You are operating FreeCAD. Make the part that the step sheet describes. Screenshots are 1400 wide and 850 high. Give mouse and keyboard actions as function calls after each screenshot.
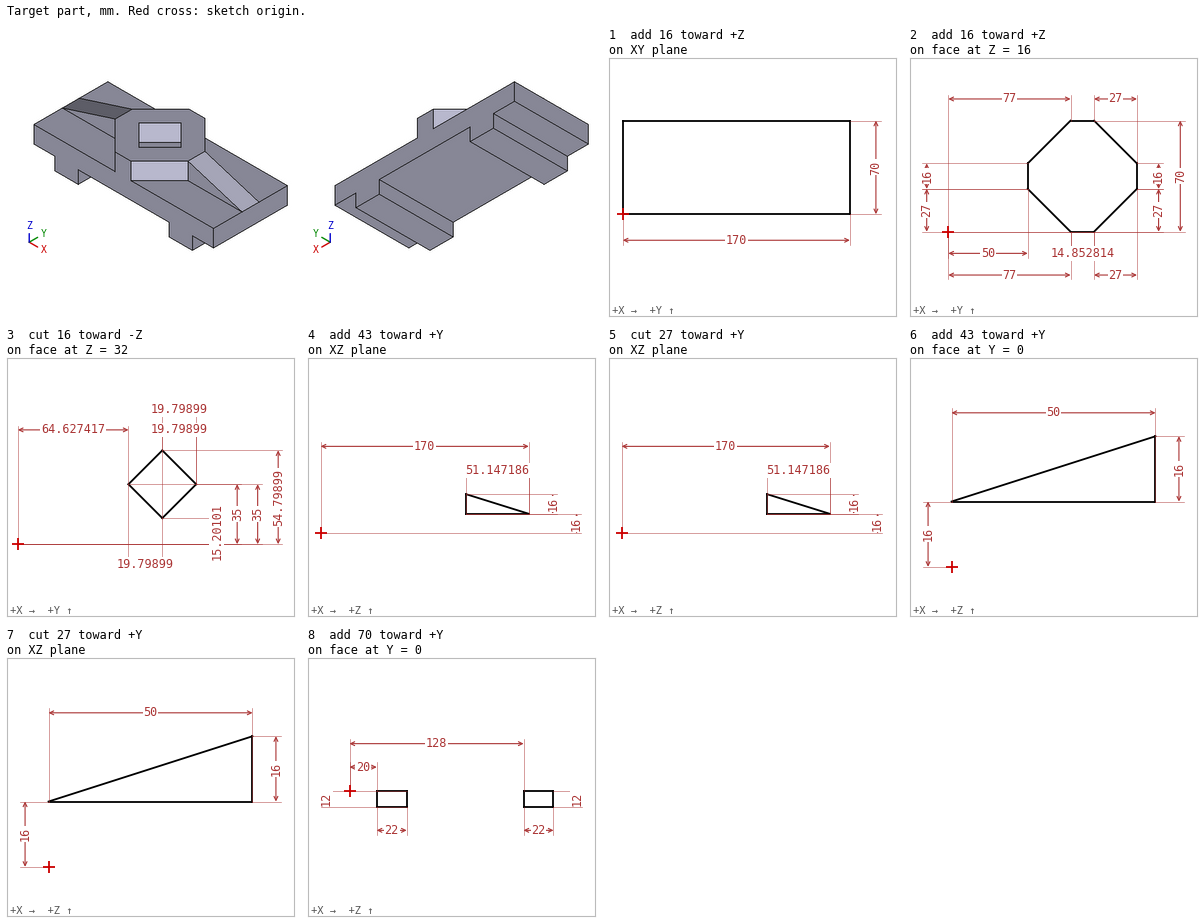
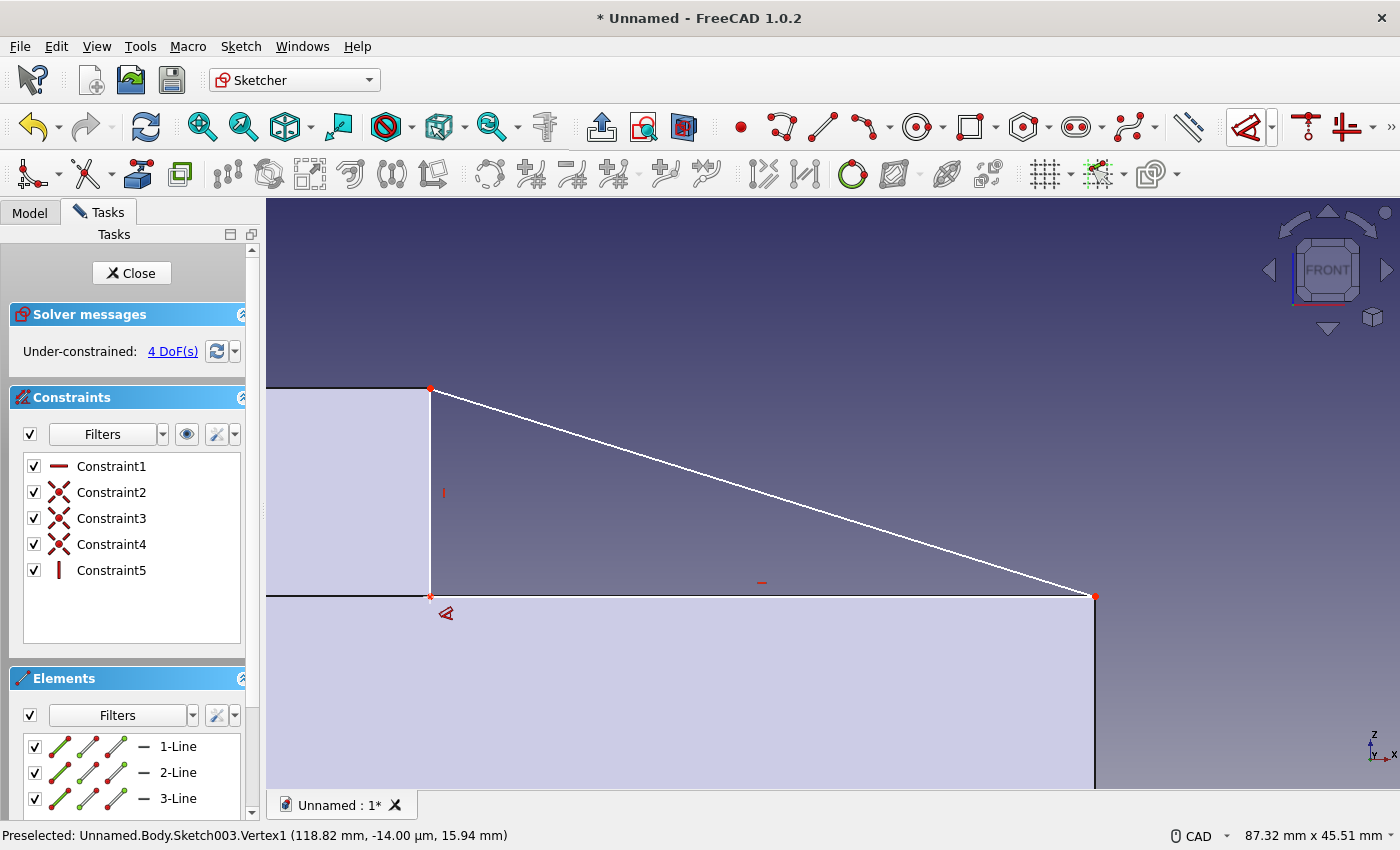
click(430, 451)
click(396, 493)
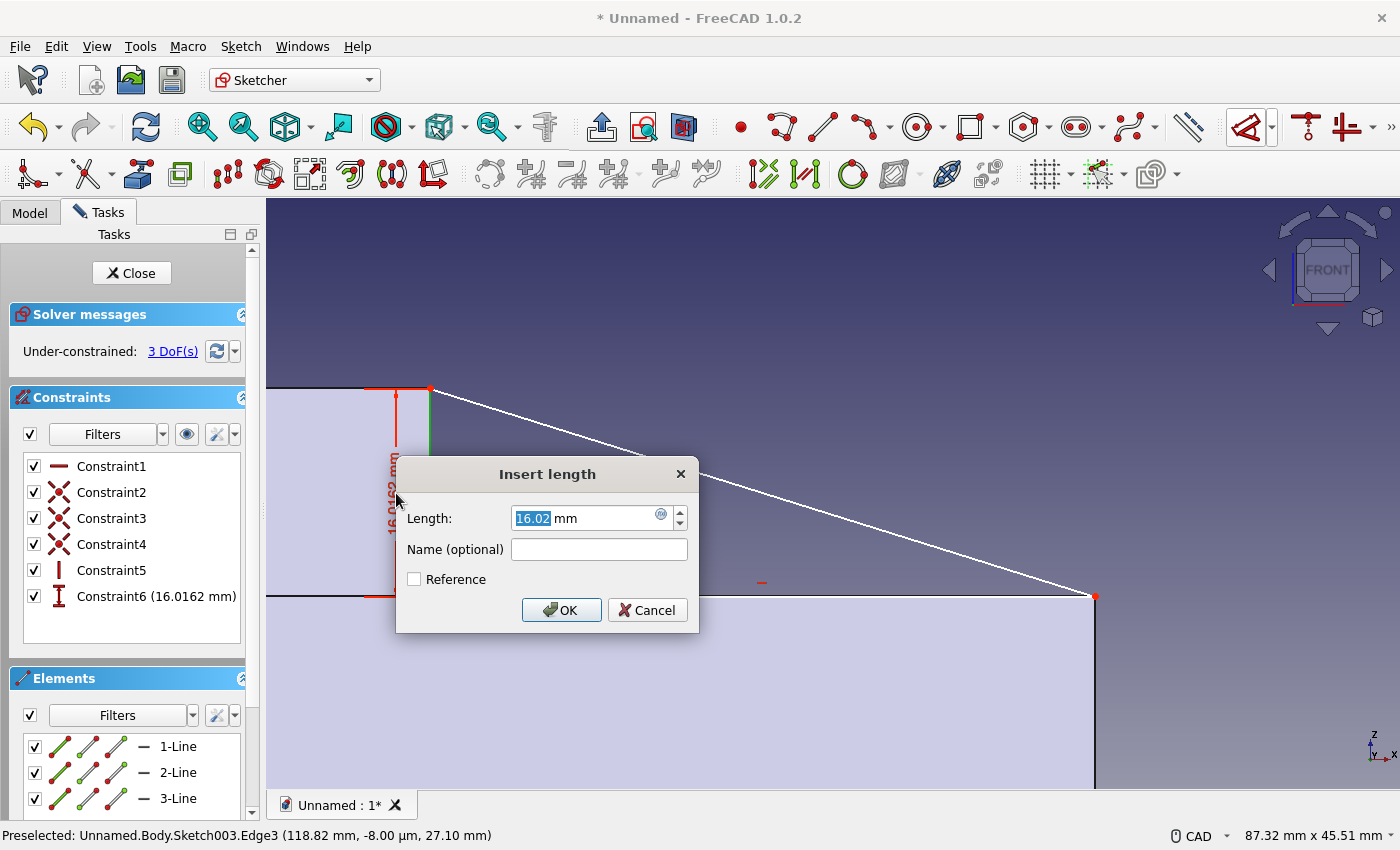
text(16)
key(Return)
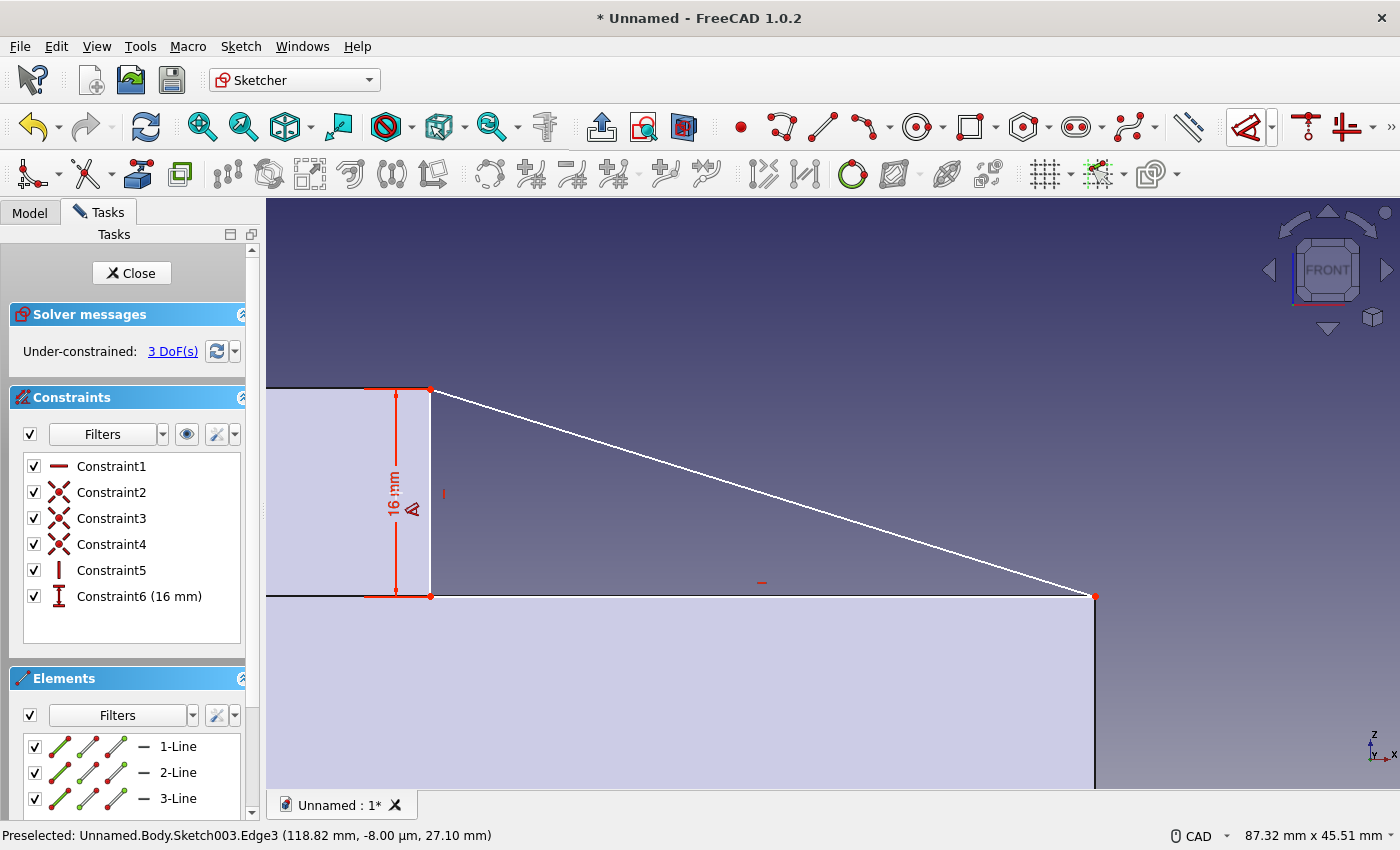
click(430, 597)
click(464, 679)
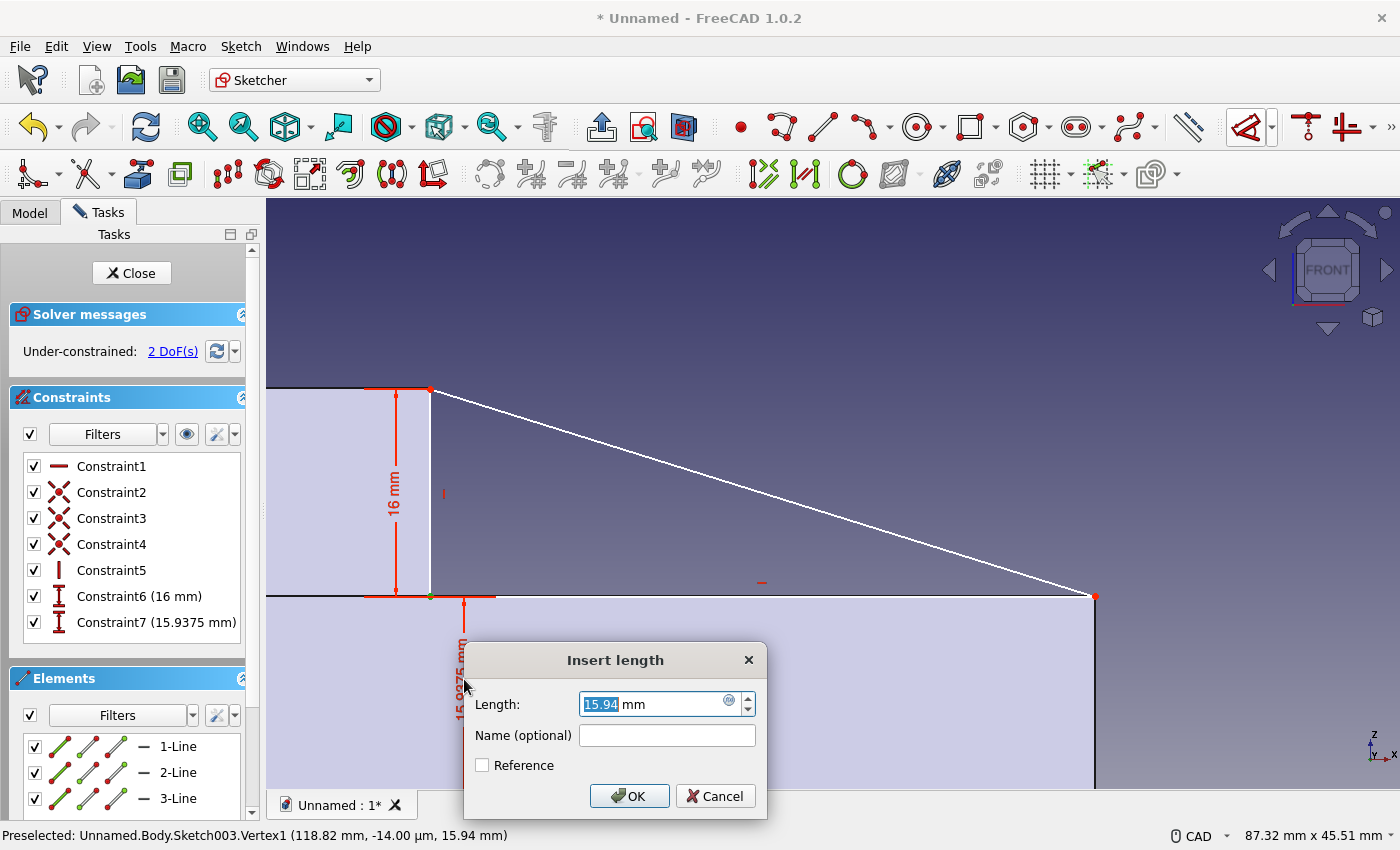
text(16)
key(Return)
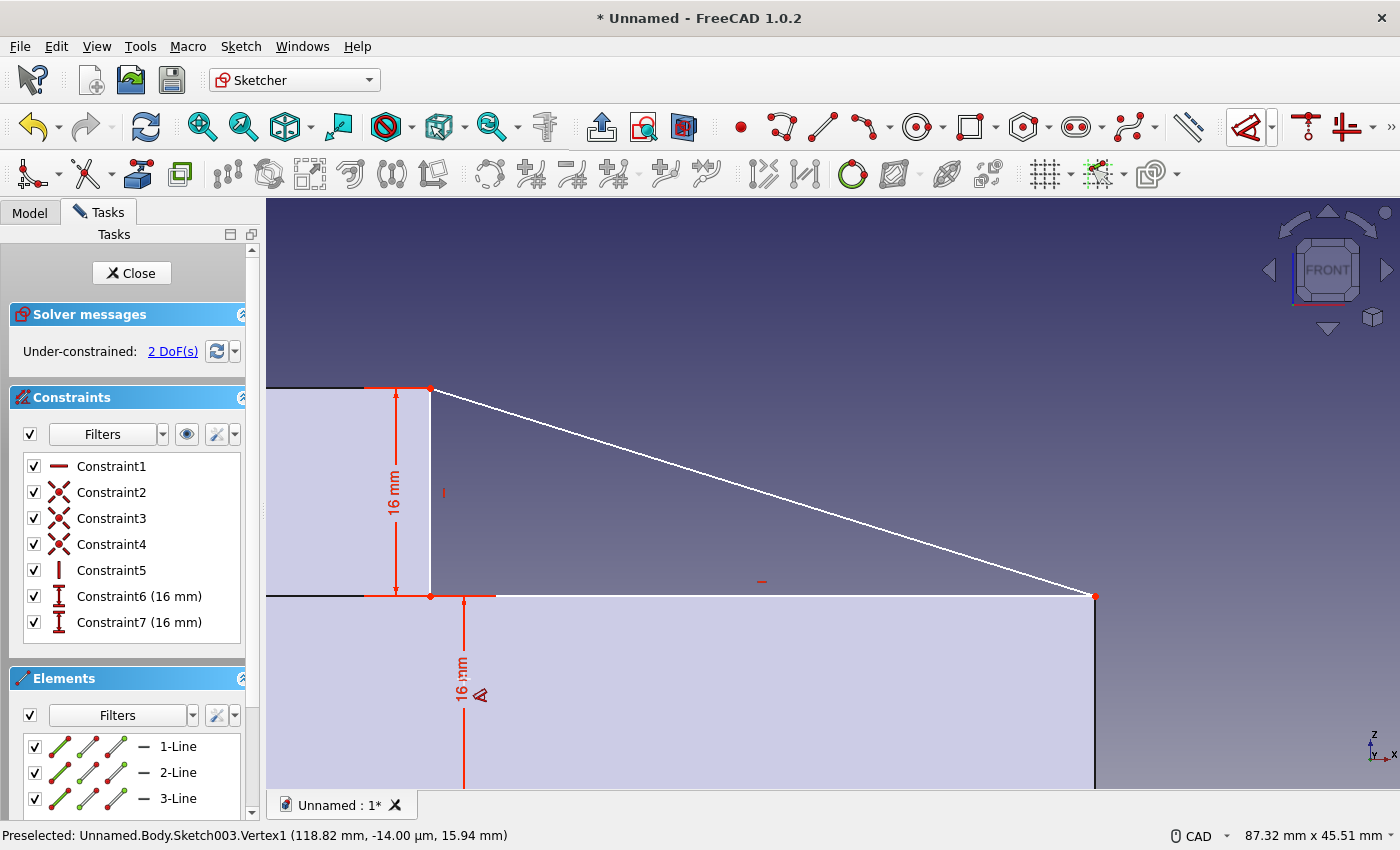
click(1095, 596)
click(695, 562)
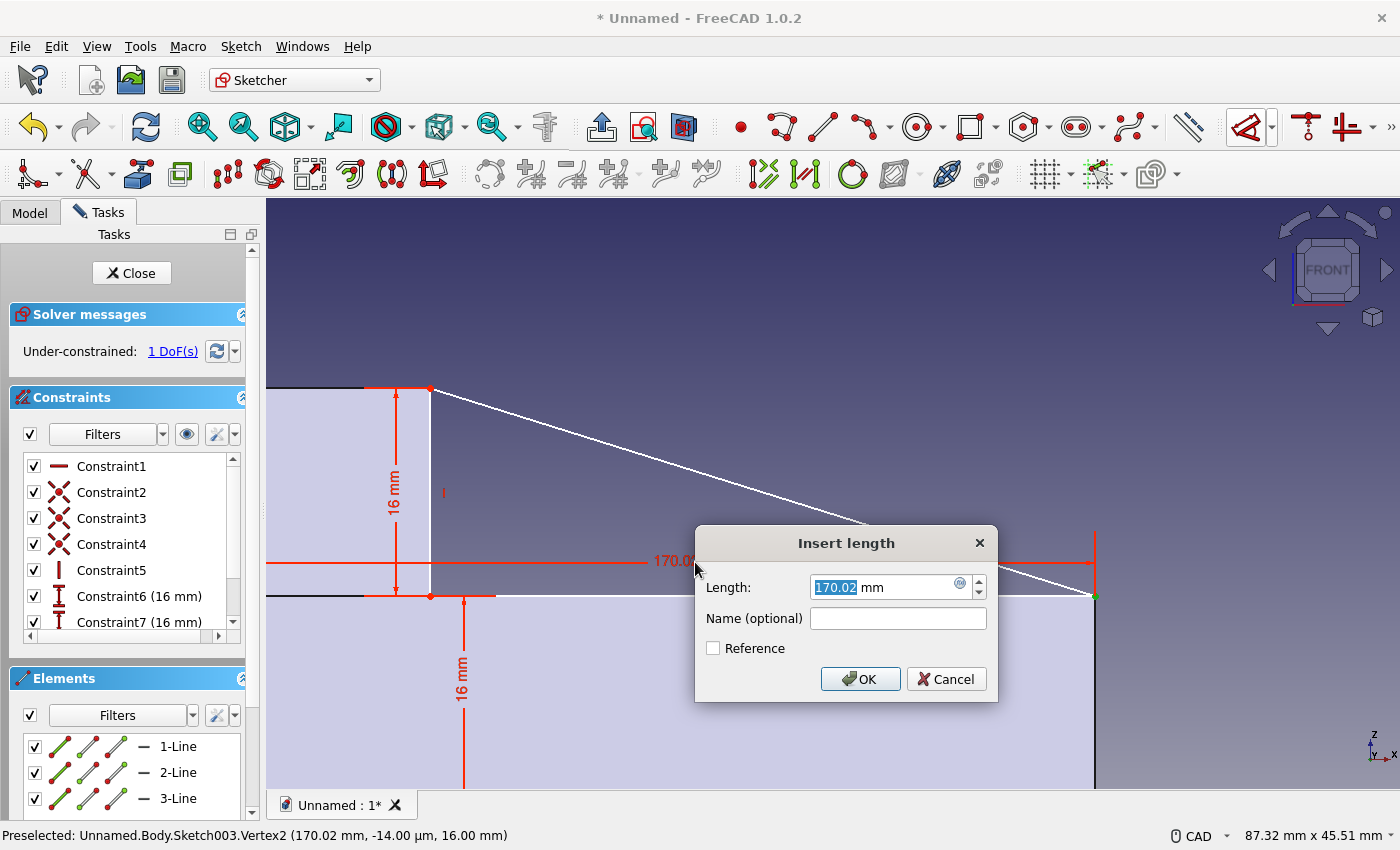
text(170)
key(Return)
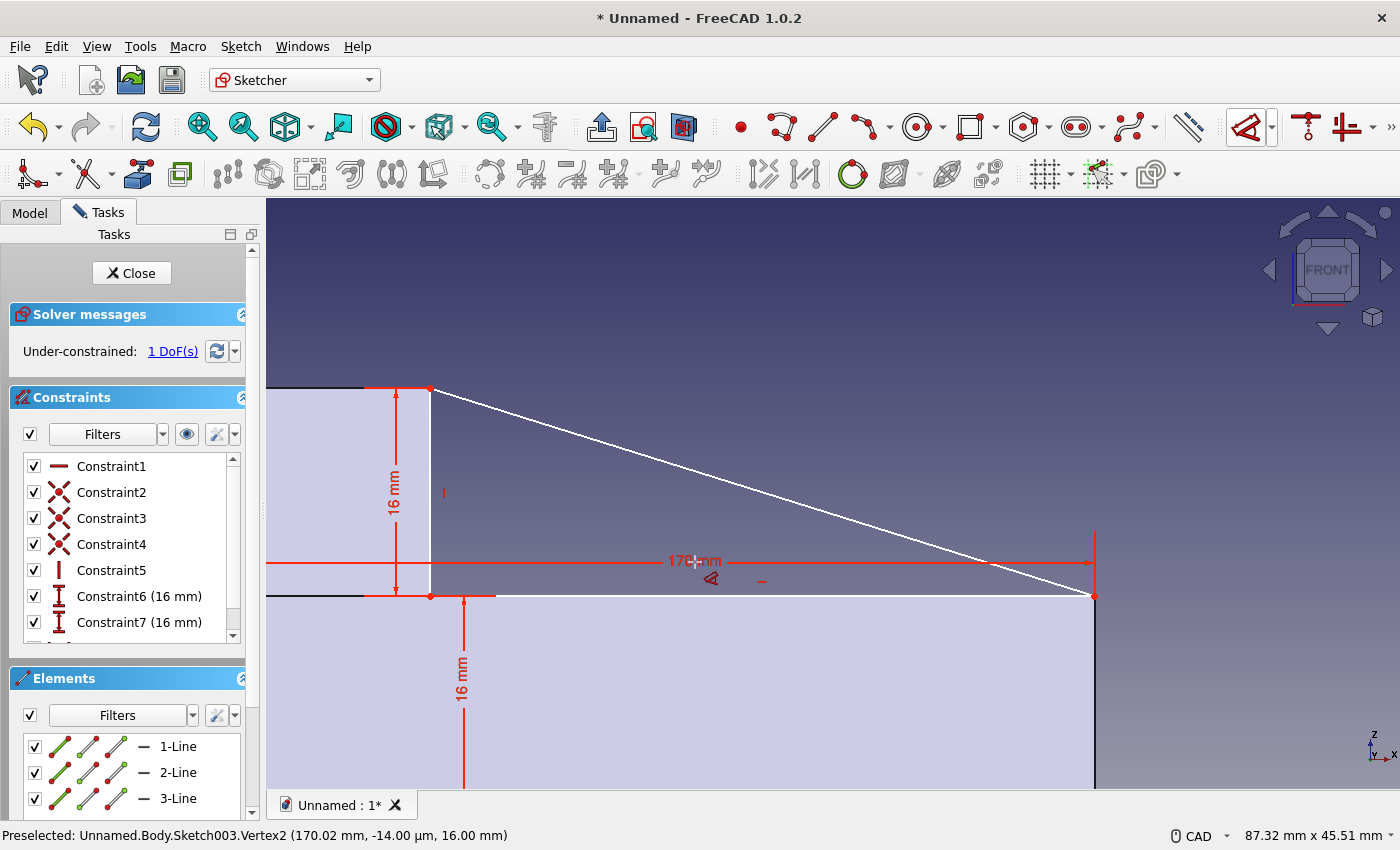
click(629, 596)
click(762, 630)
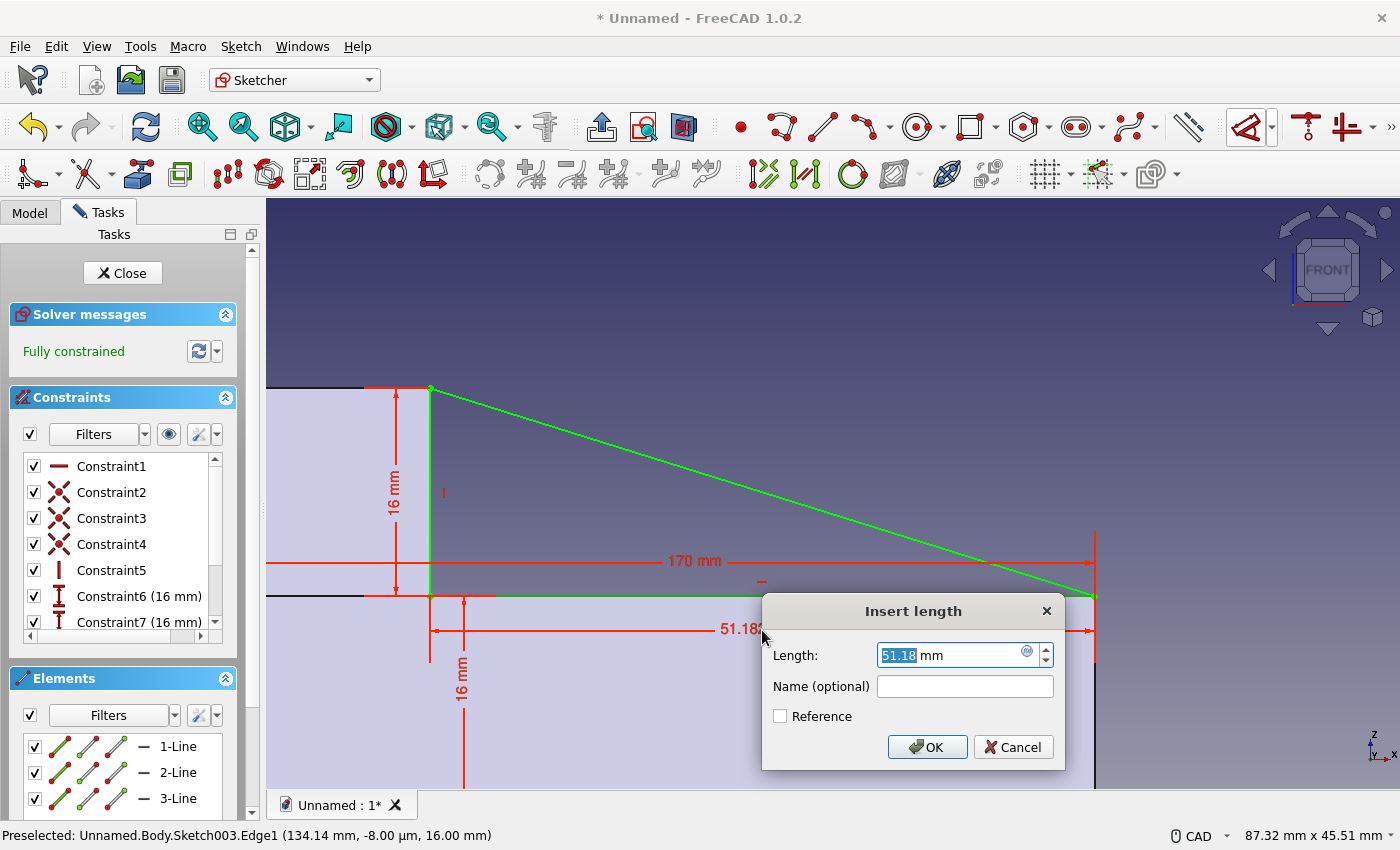
text(51.147186)
key(Return)
key(Escape)